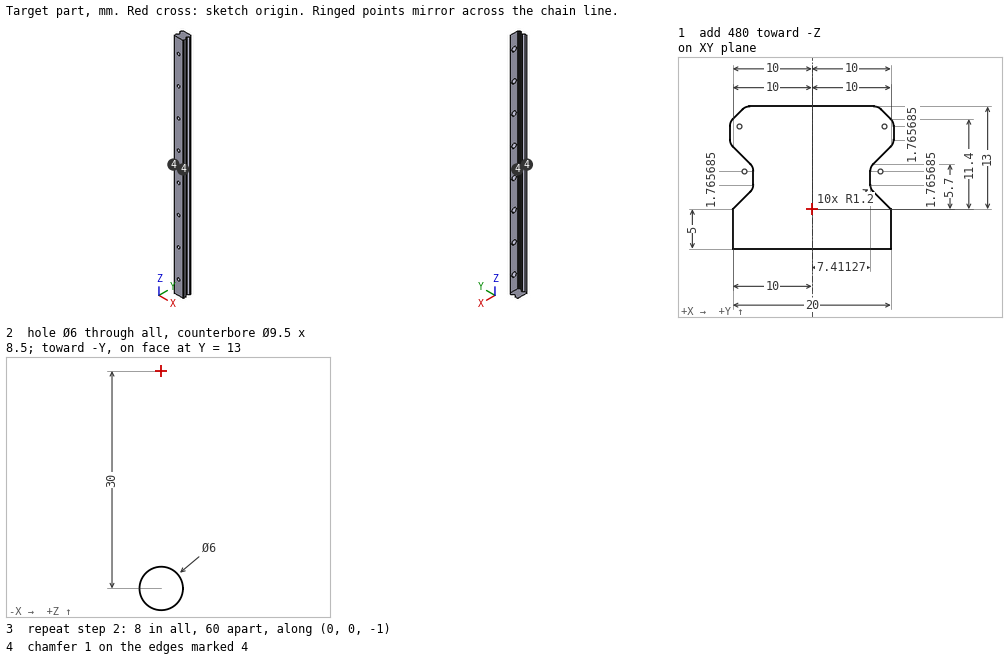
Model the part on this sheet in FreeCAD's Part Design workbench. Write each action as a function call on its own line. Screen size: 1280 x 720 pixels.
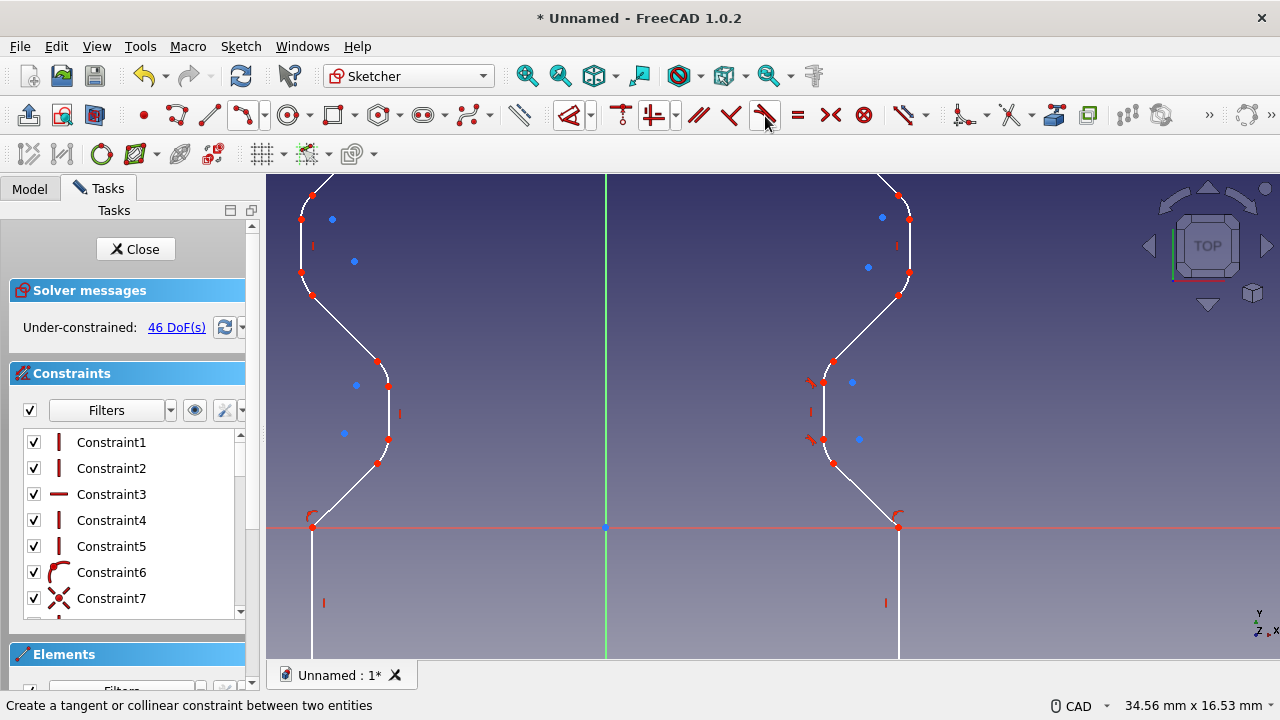
click(853, 342)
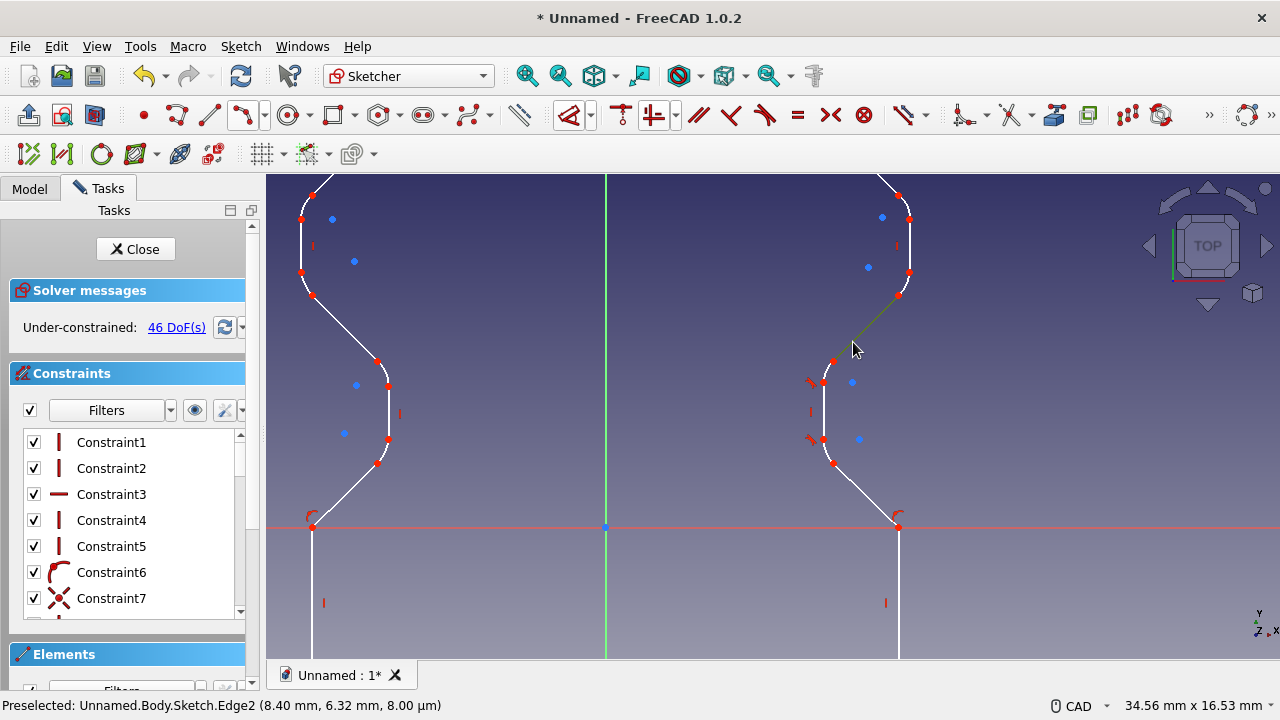
click(826, 371)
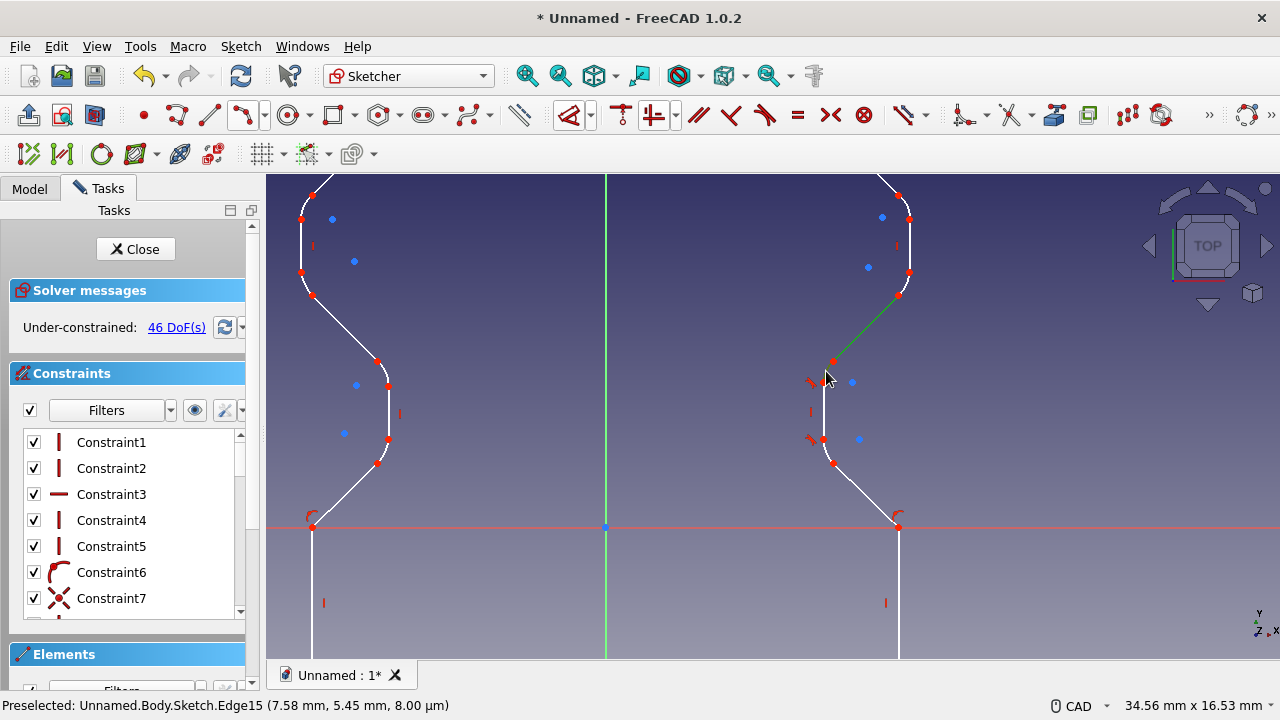
click(765, 116)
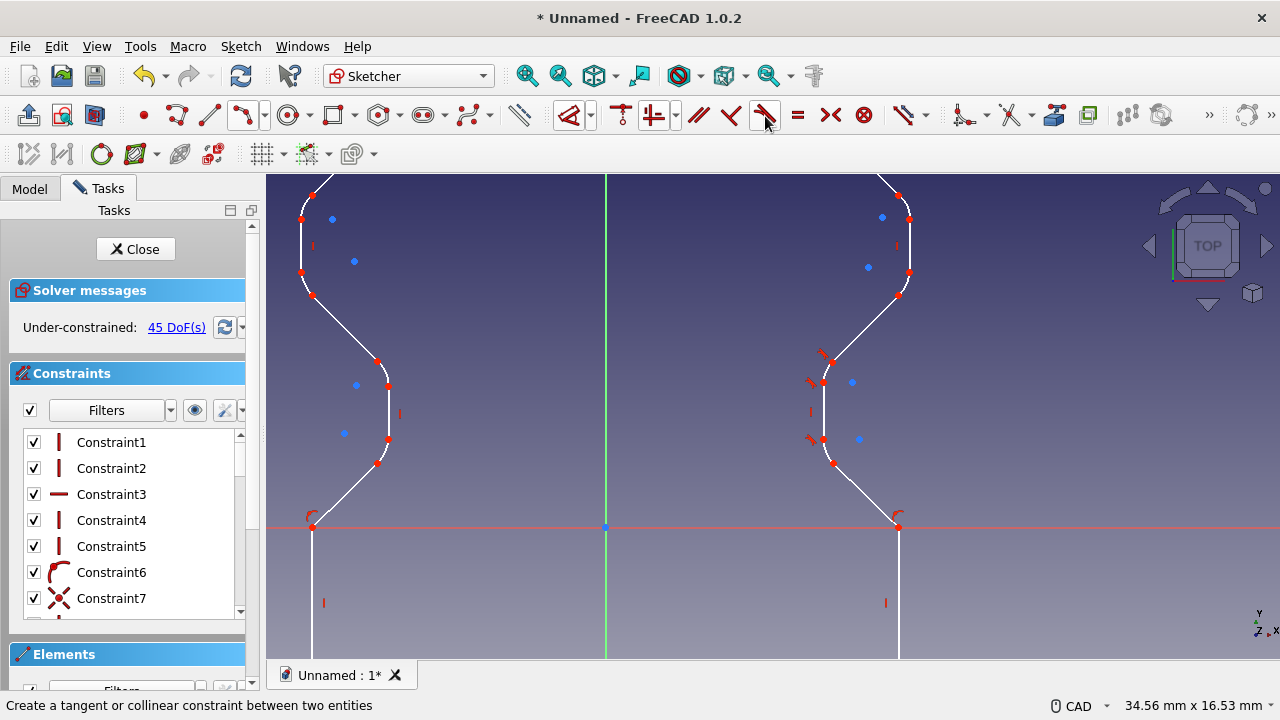
click(852, 342)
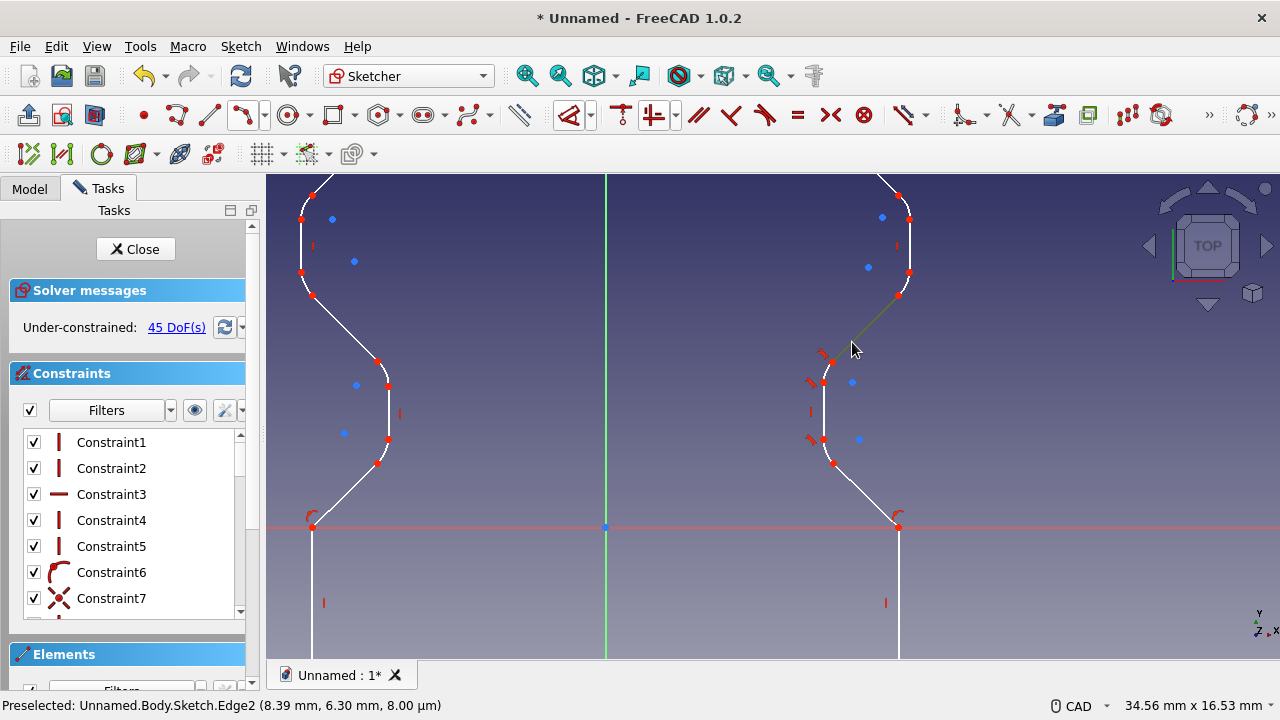
click(906, 285)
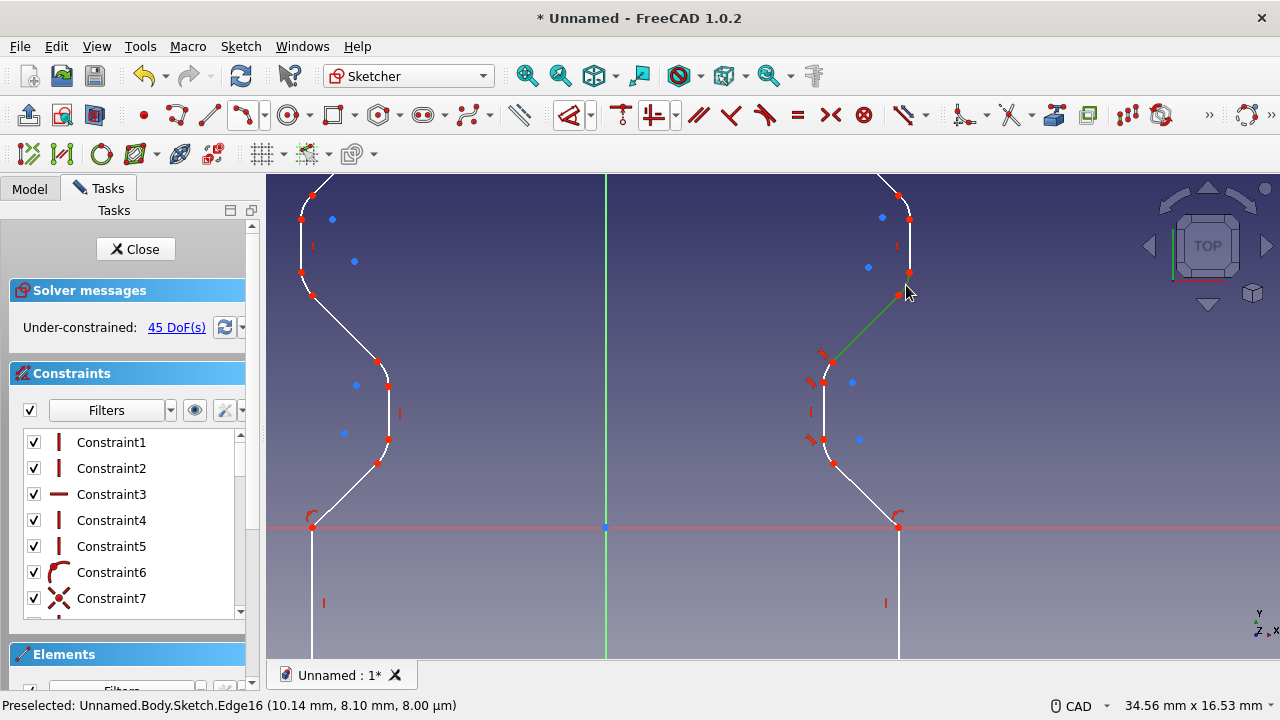
click(765, 116)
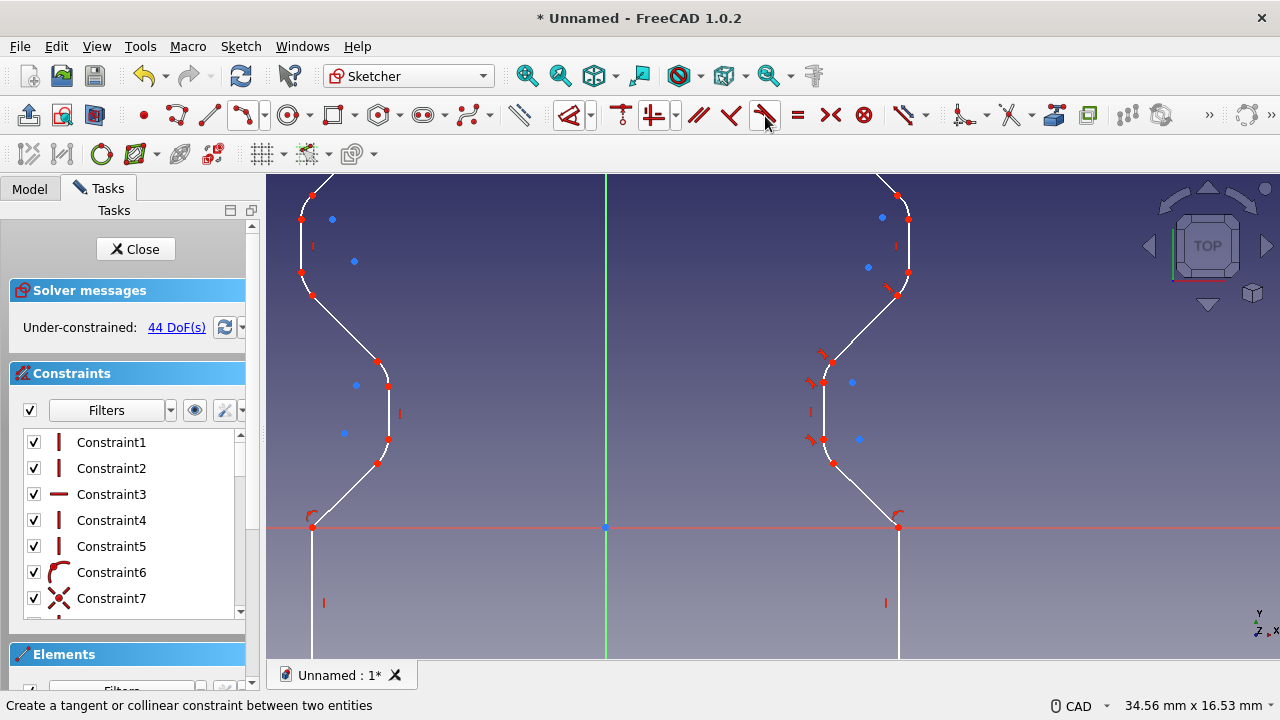
click(909, 256)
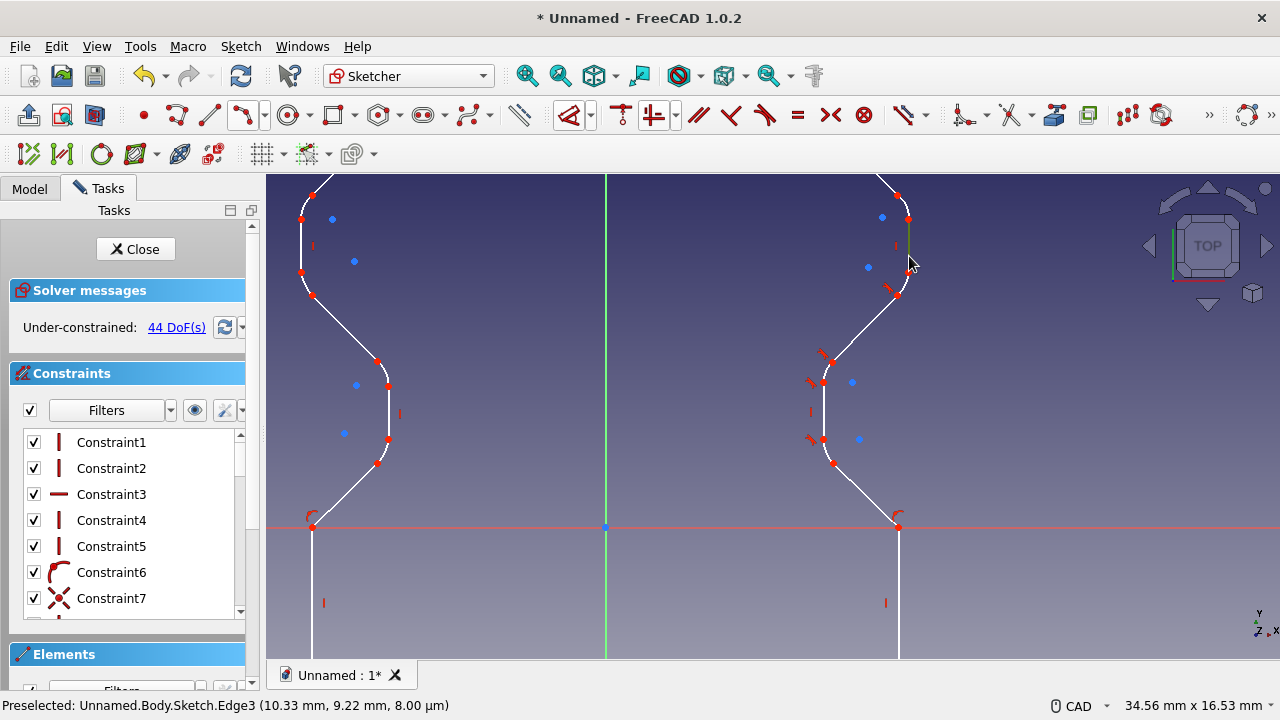
click(905, 285)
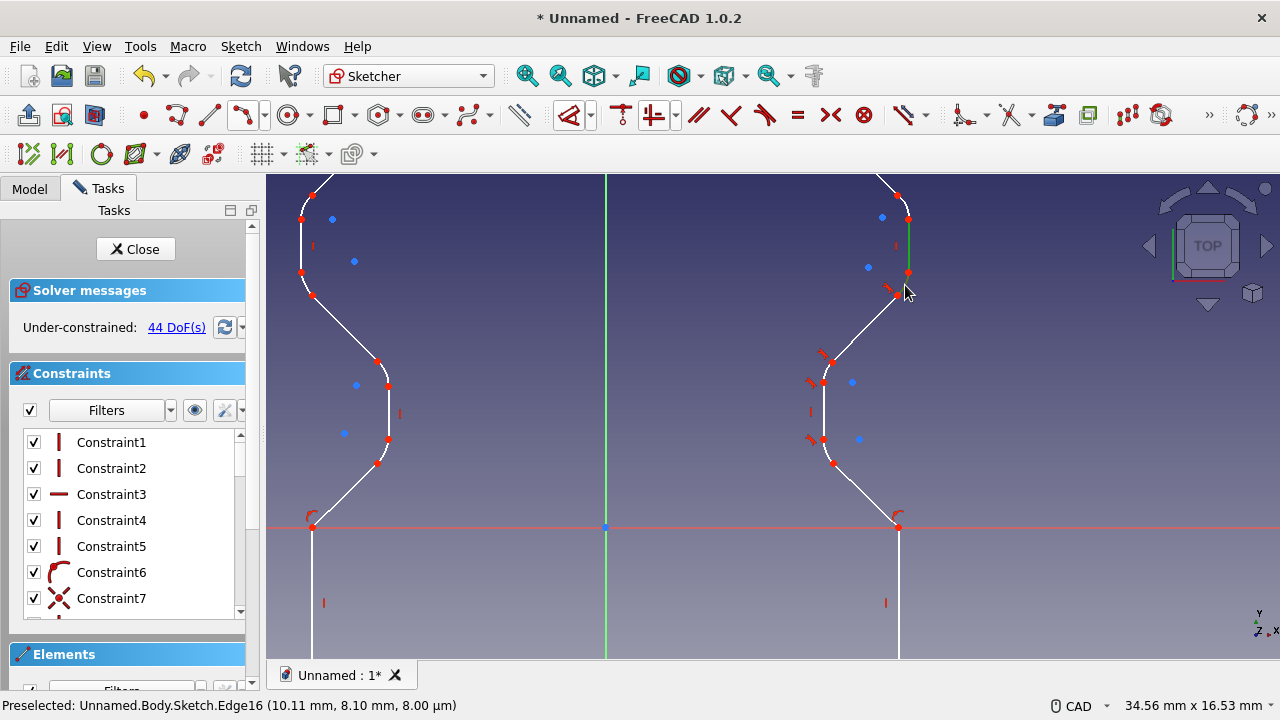
key(t)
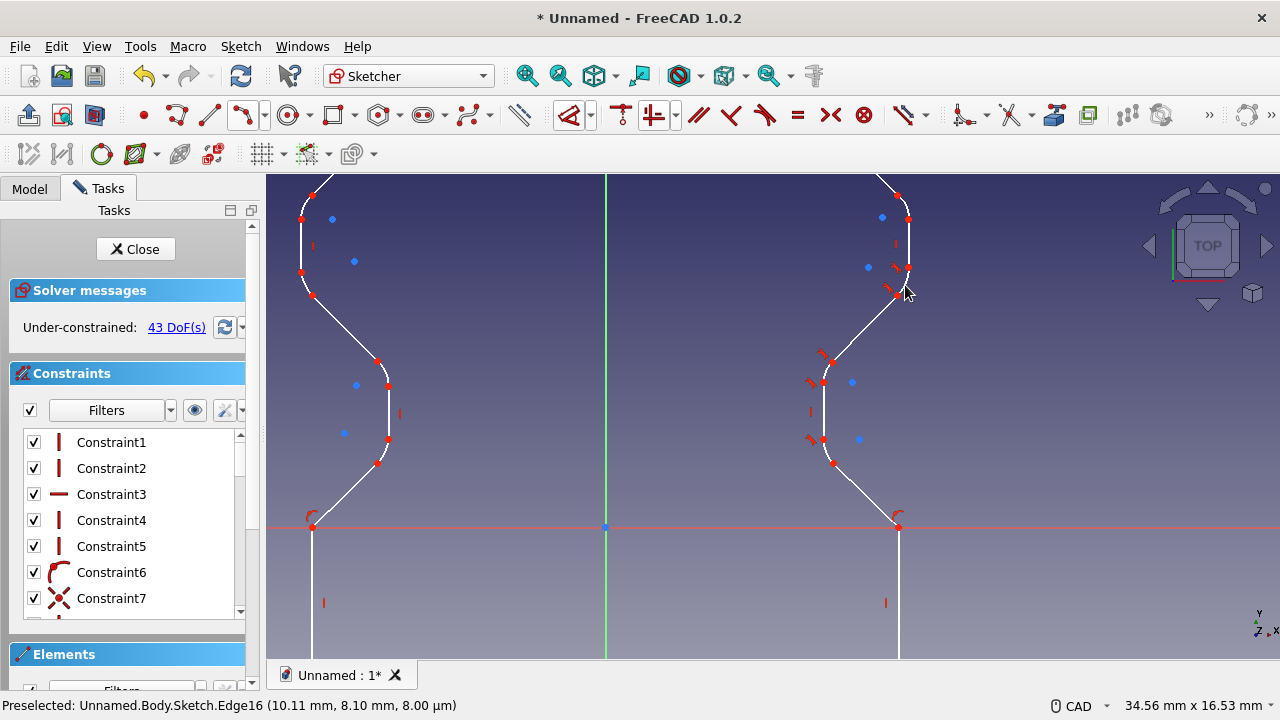
click(909, 253)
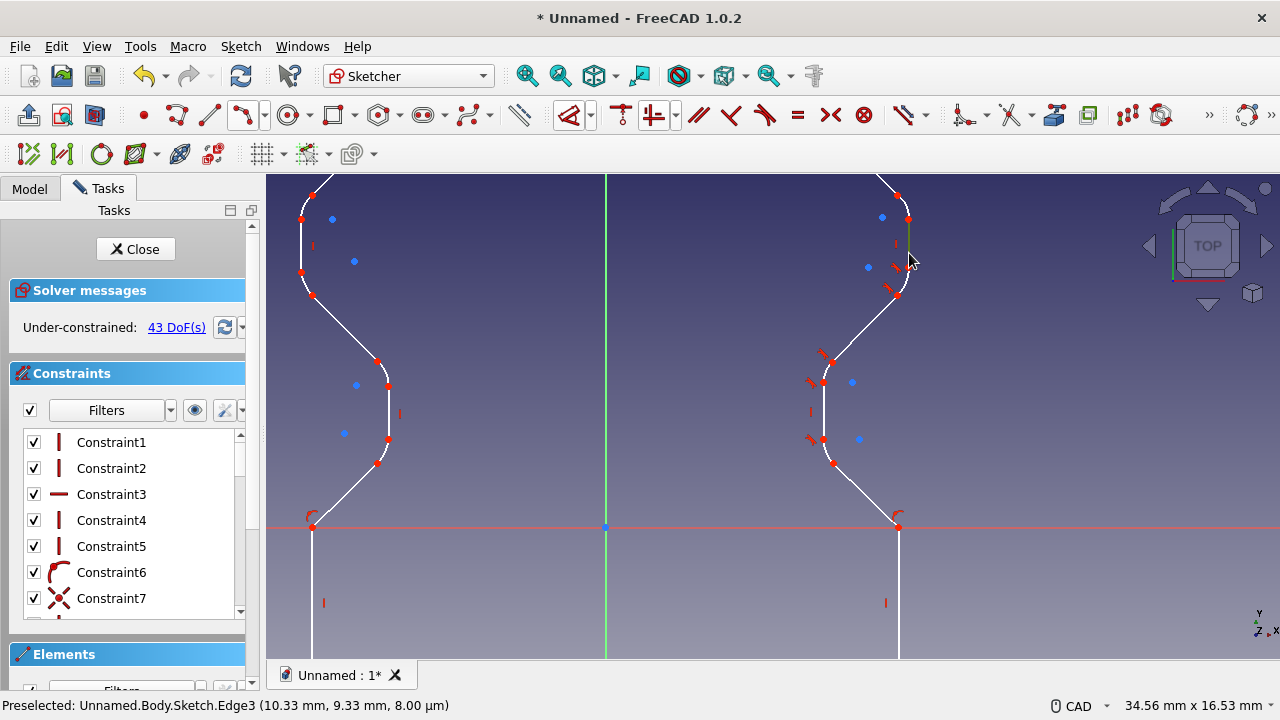
click(906, 206)